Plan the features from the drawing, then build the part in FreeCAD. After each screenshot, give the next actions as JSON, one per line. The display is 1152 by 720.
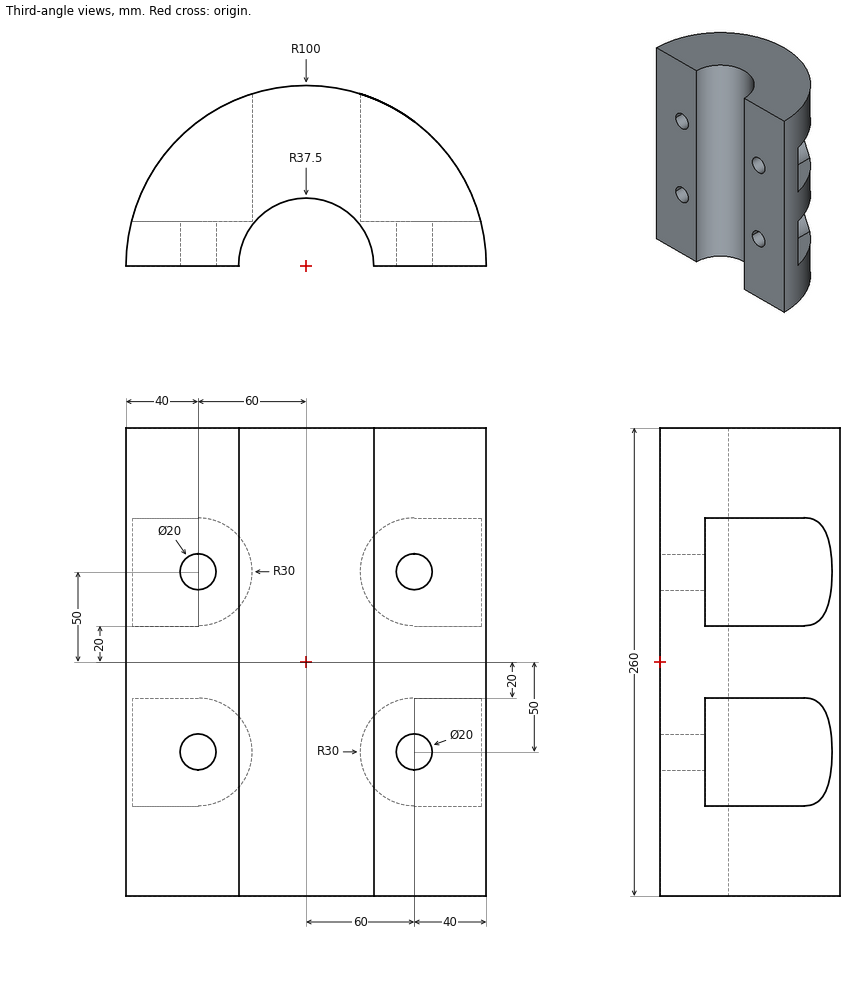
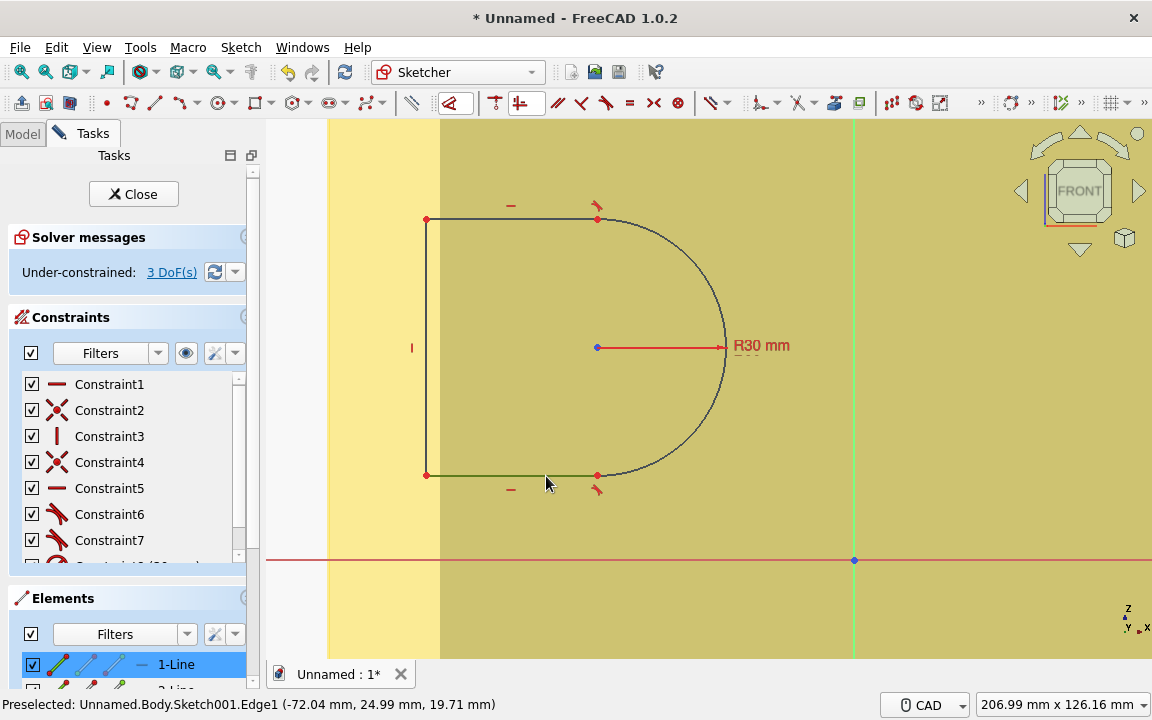
{"action": "key", "text": "l"}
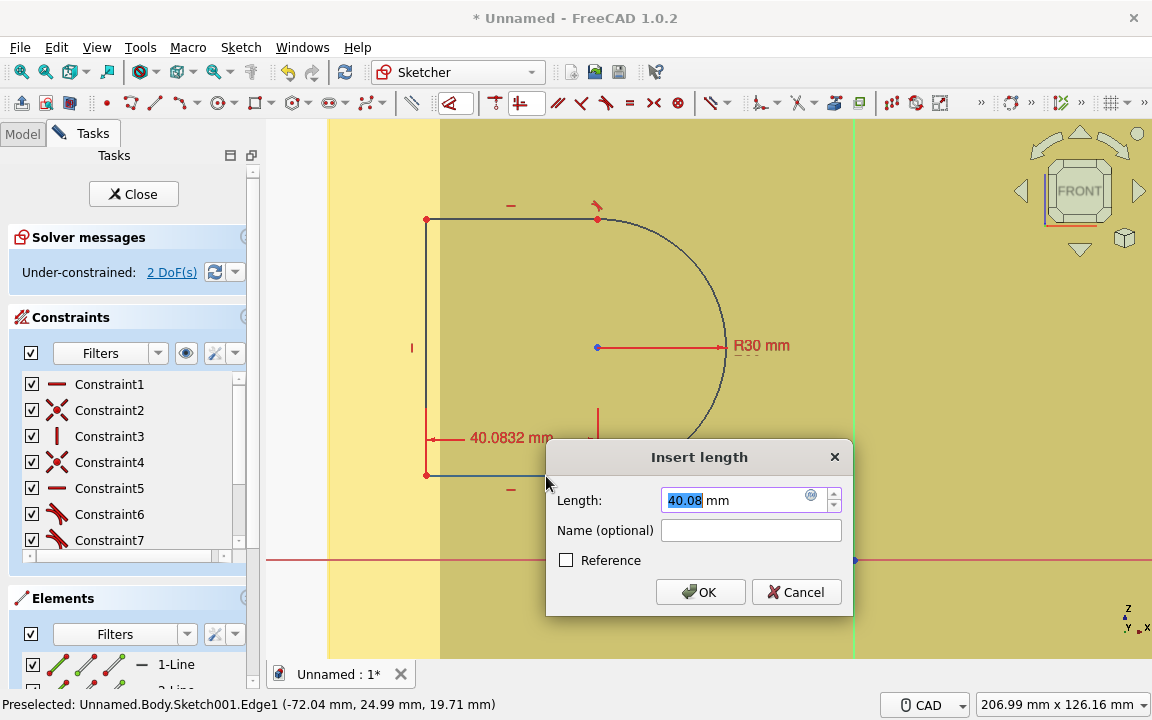
{"action": "type", "text": "40"}
{"action": "key", "text": "Return"}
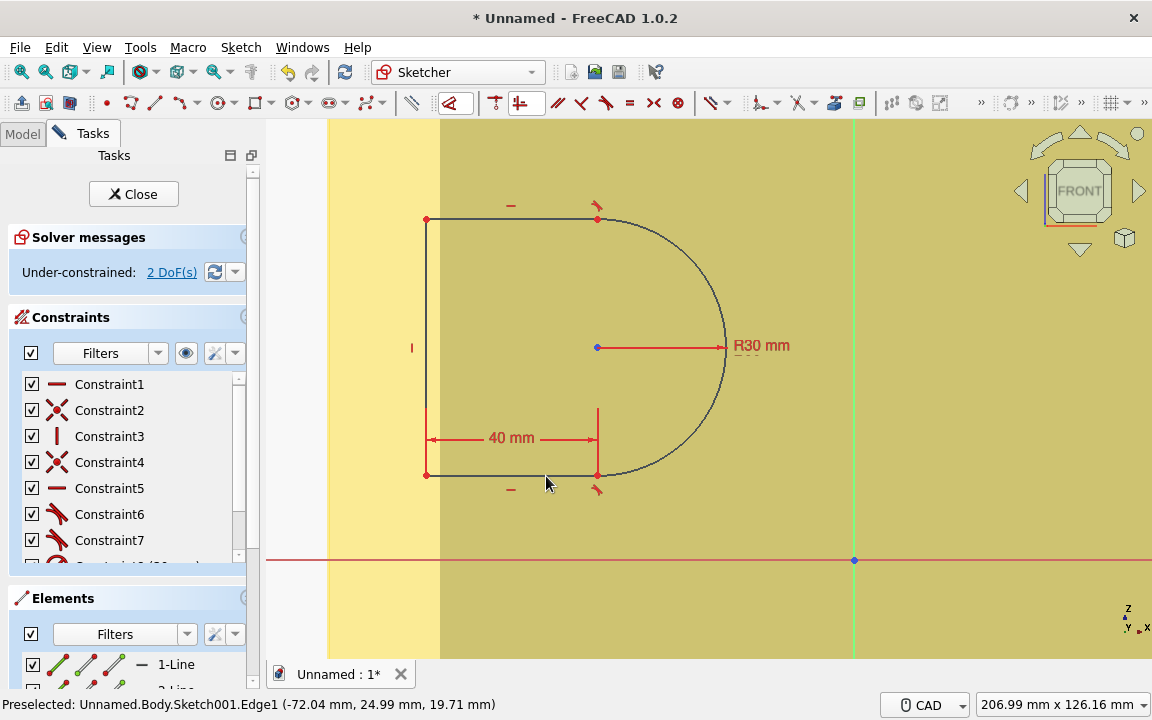
{"action": "left_click", "coordinate": [598, 476]}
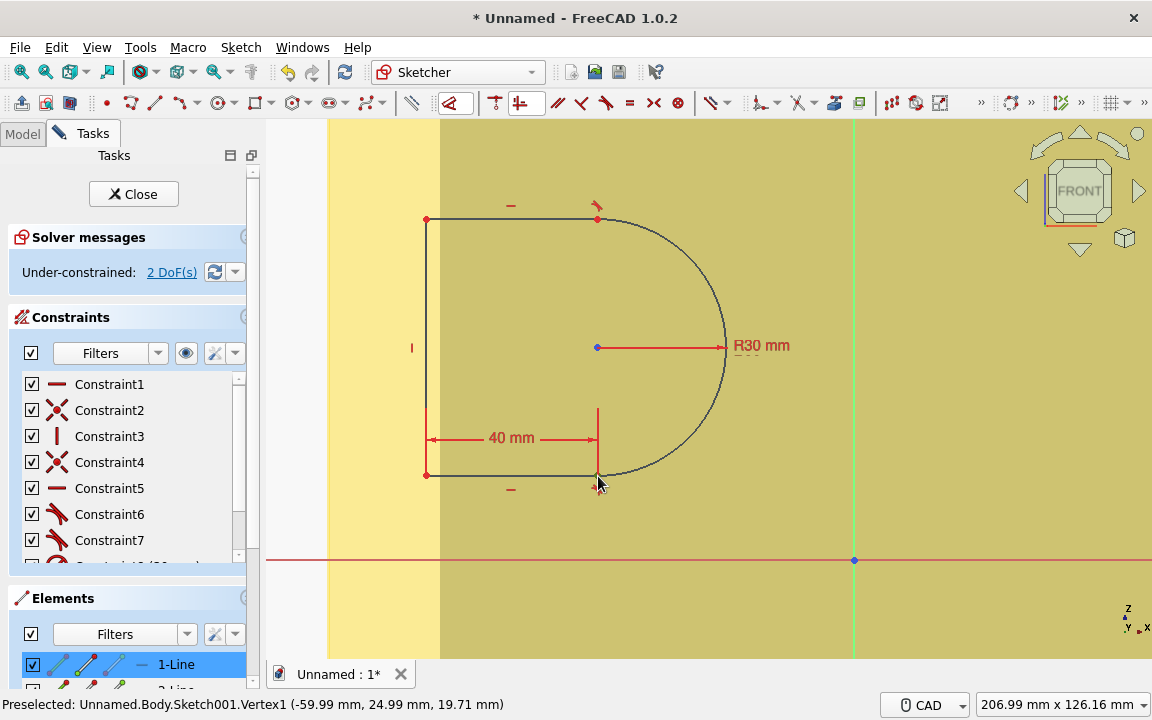
{"action": "left_click", "coordinate": [468, 104]}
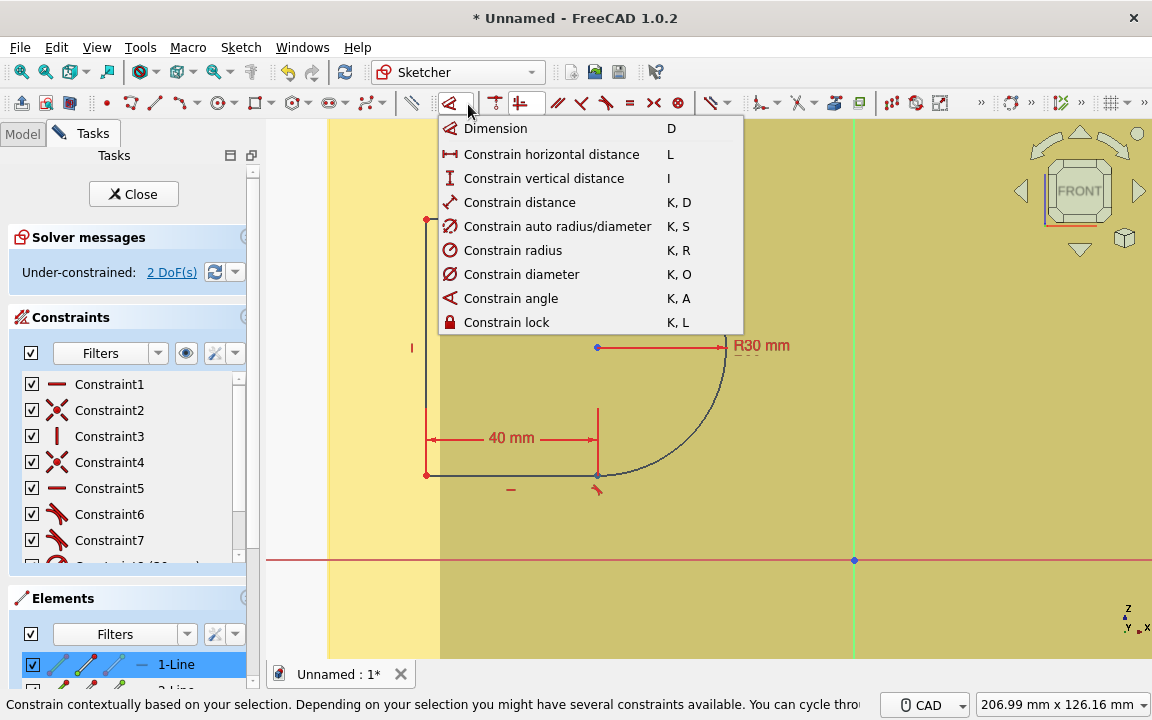
{"action": "left_click", "coordinate": [591, 154]}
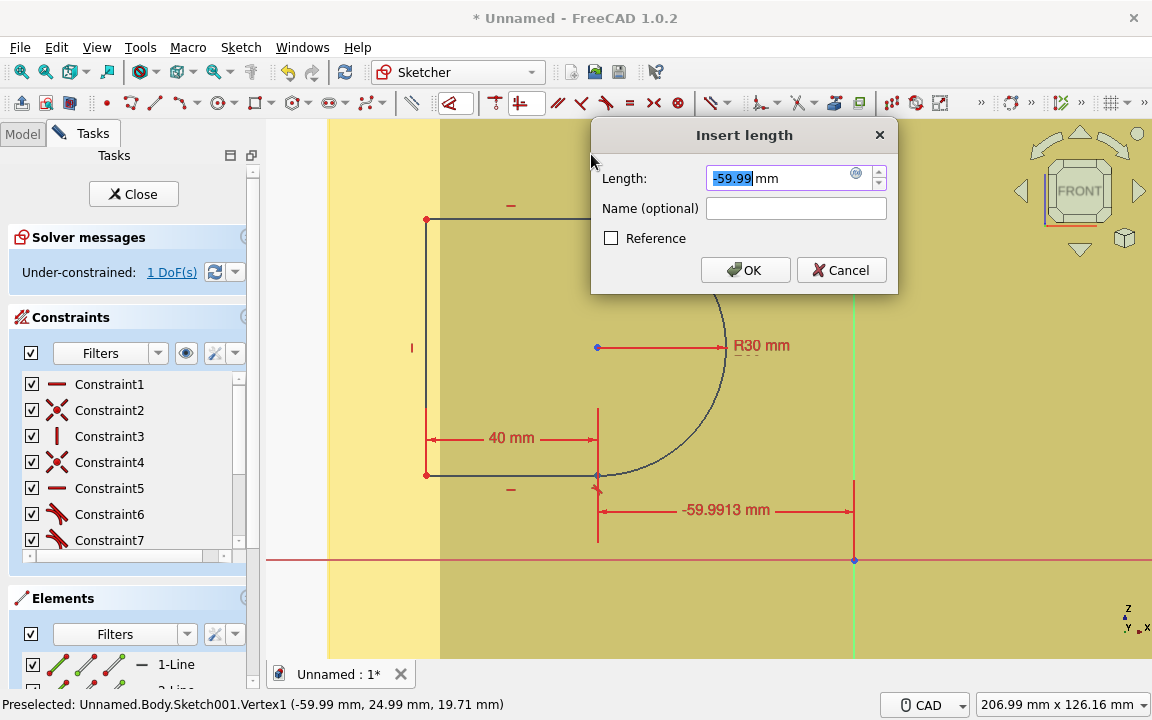
{"action": "type", "text": "-60"}
{"action": "key", "text": "Return"}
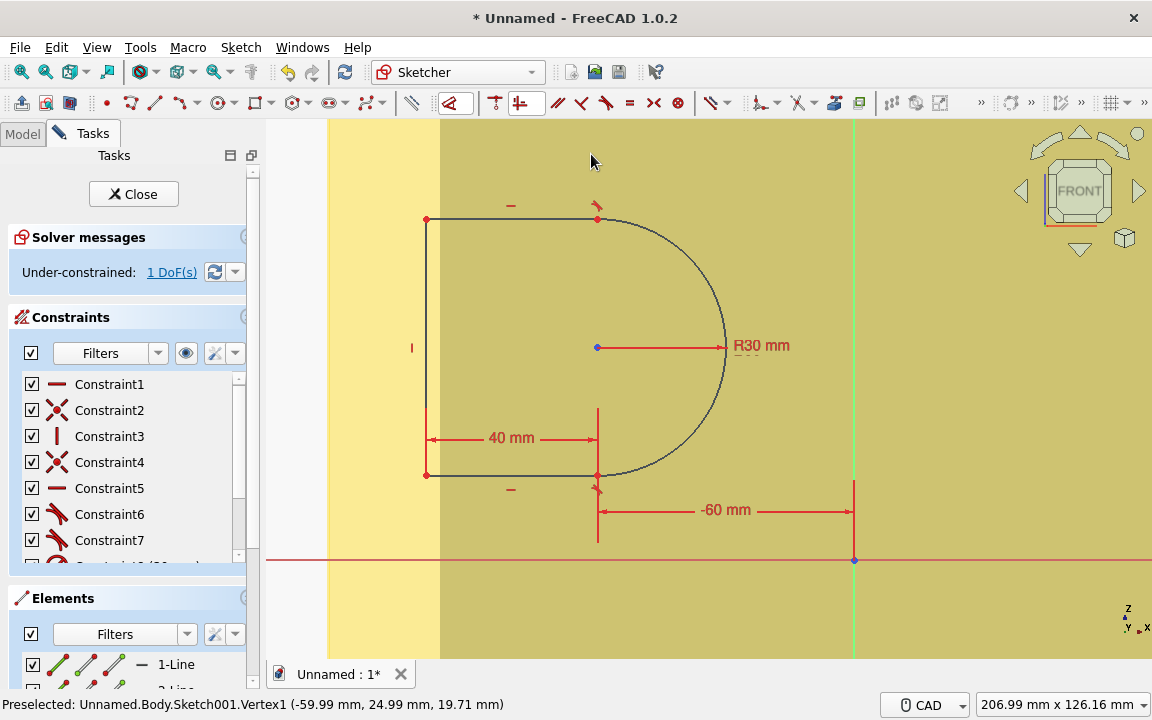
{"action": "left_click", "coordinate": [598, 476]}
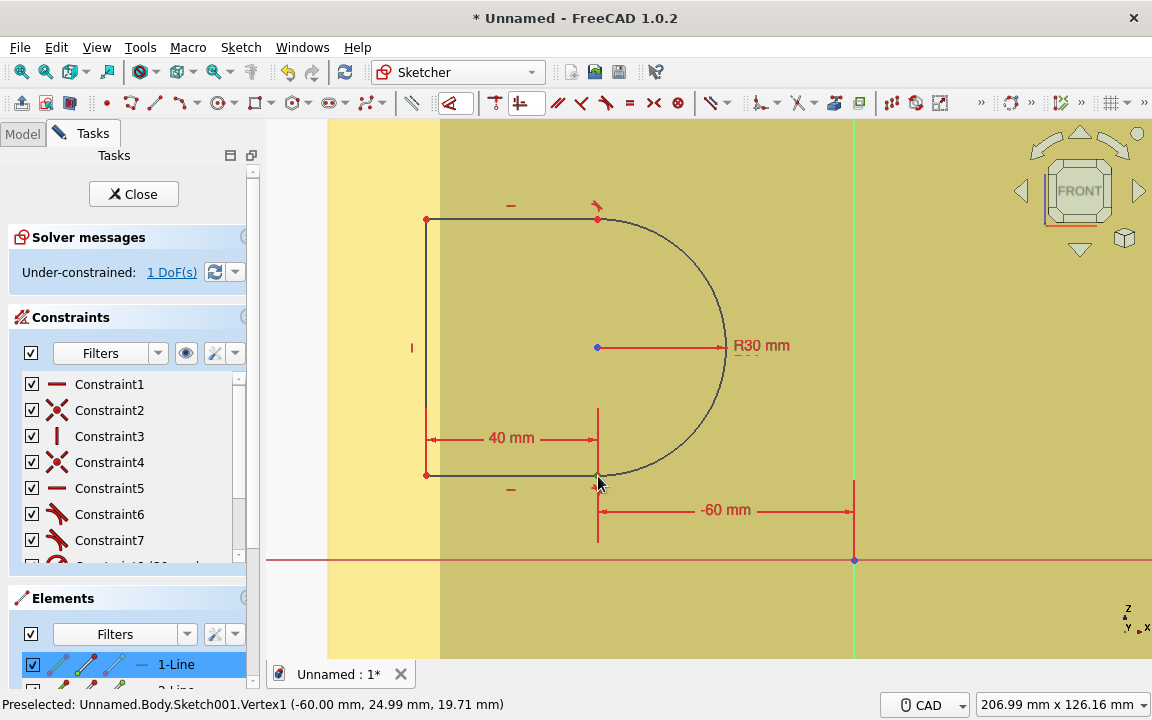
{"action": "key", "text": "i"}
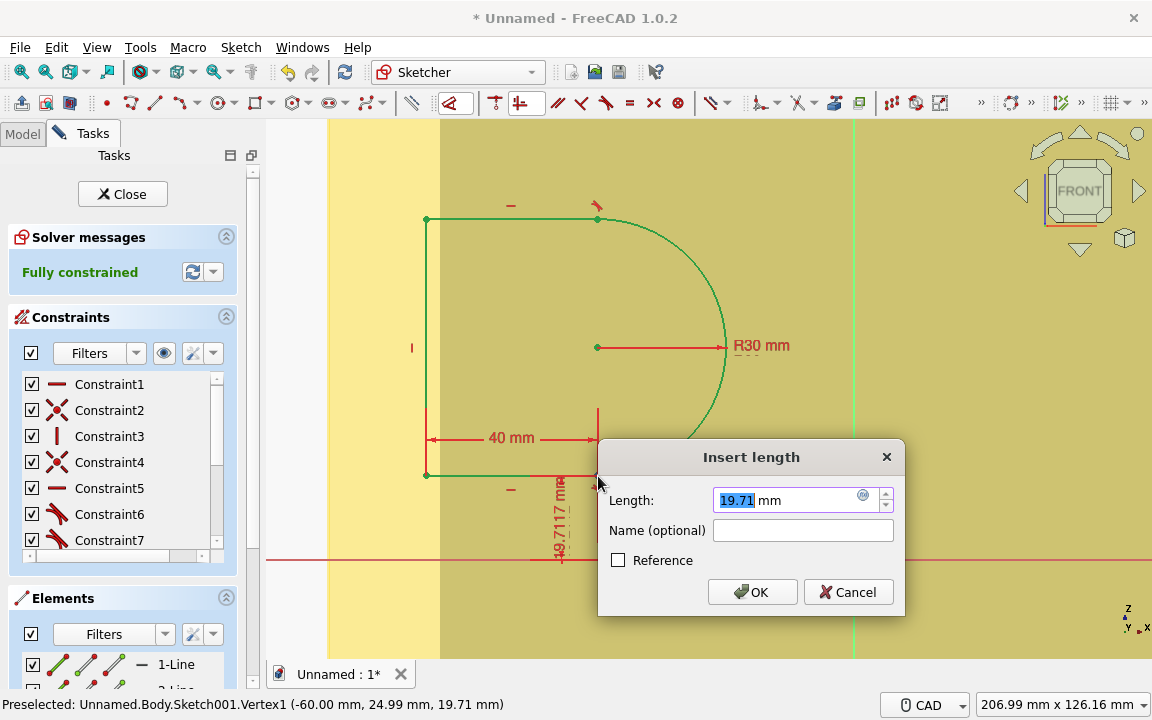
{"action": "type", "text": "20"}
{"action": "key", "text": "Return"}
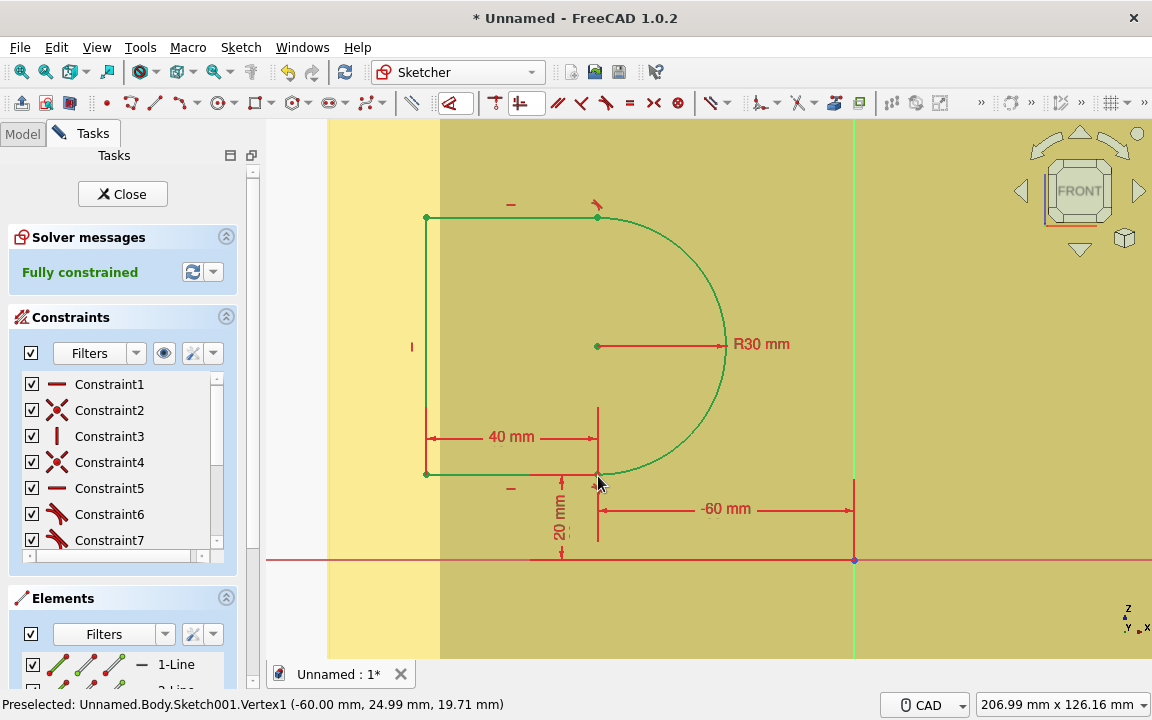
{"action": "left_click", "coordinate": [123, 194]}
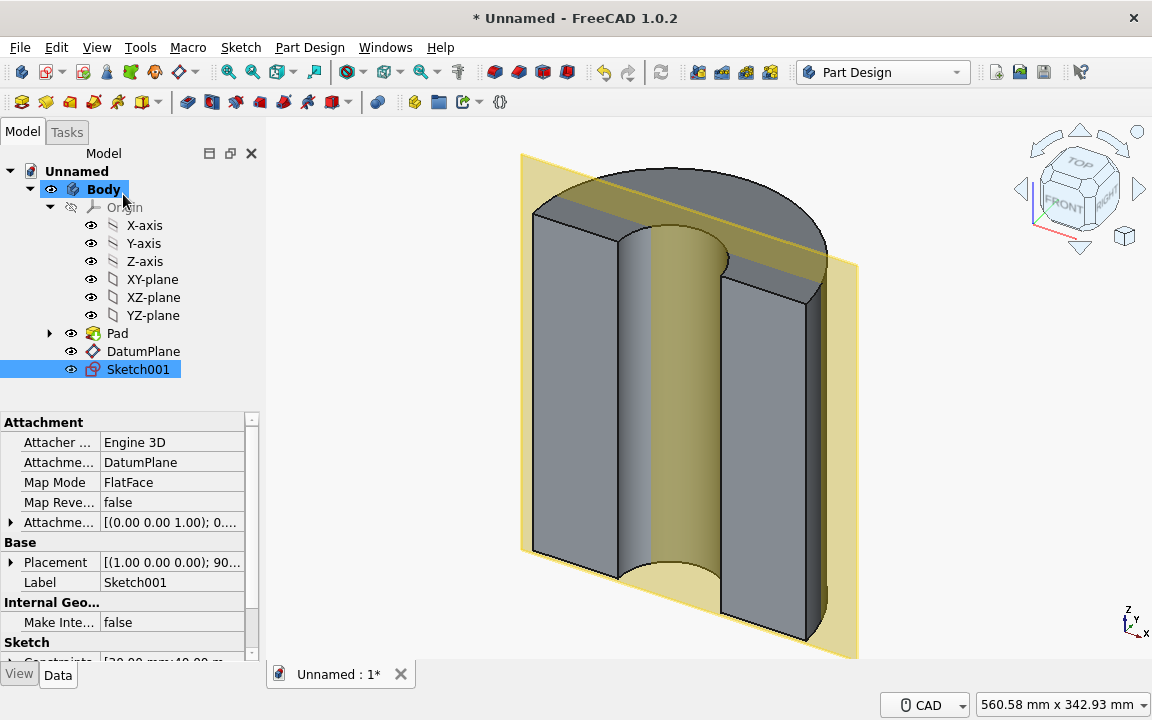
{"action": "left_click", "coordinate": [188, 102]}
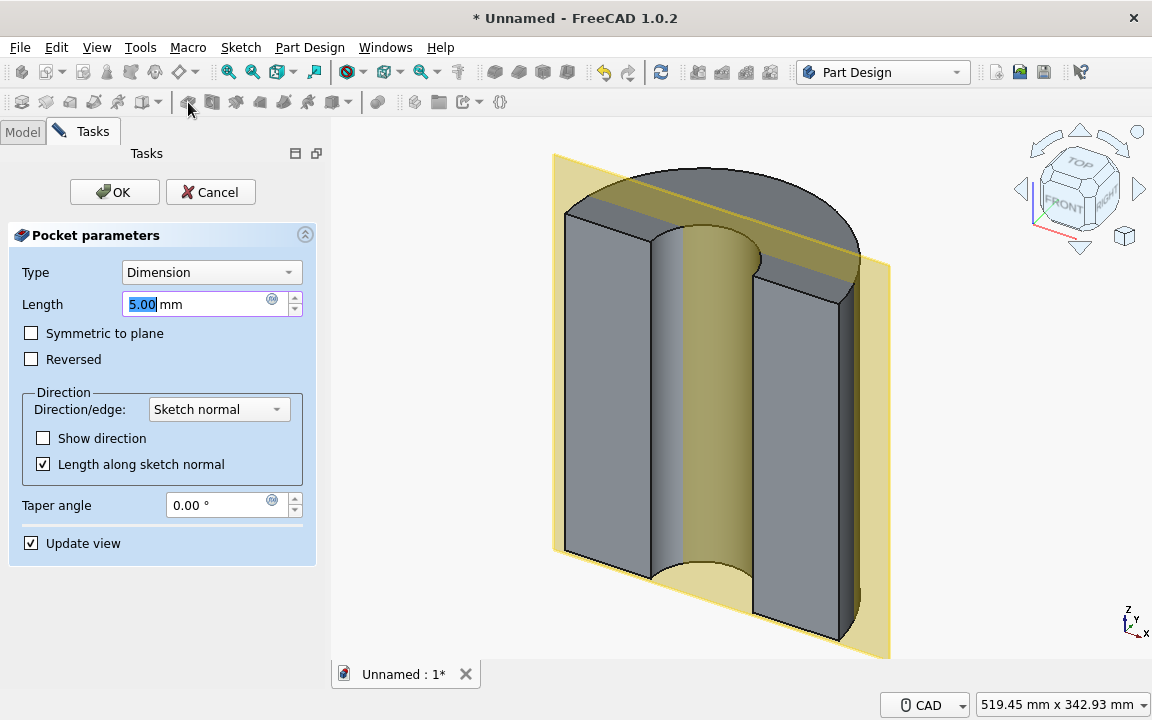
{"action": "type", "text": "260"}
{"action": "key", "text": "Tab"}